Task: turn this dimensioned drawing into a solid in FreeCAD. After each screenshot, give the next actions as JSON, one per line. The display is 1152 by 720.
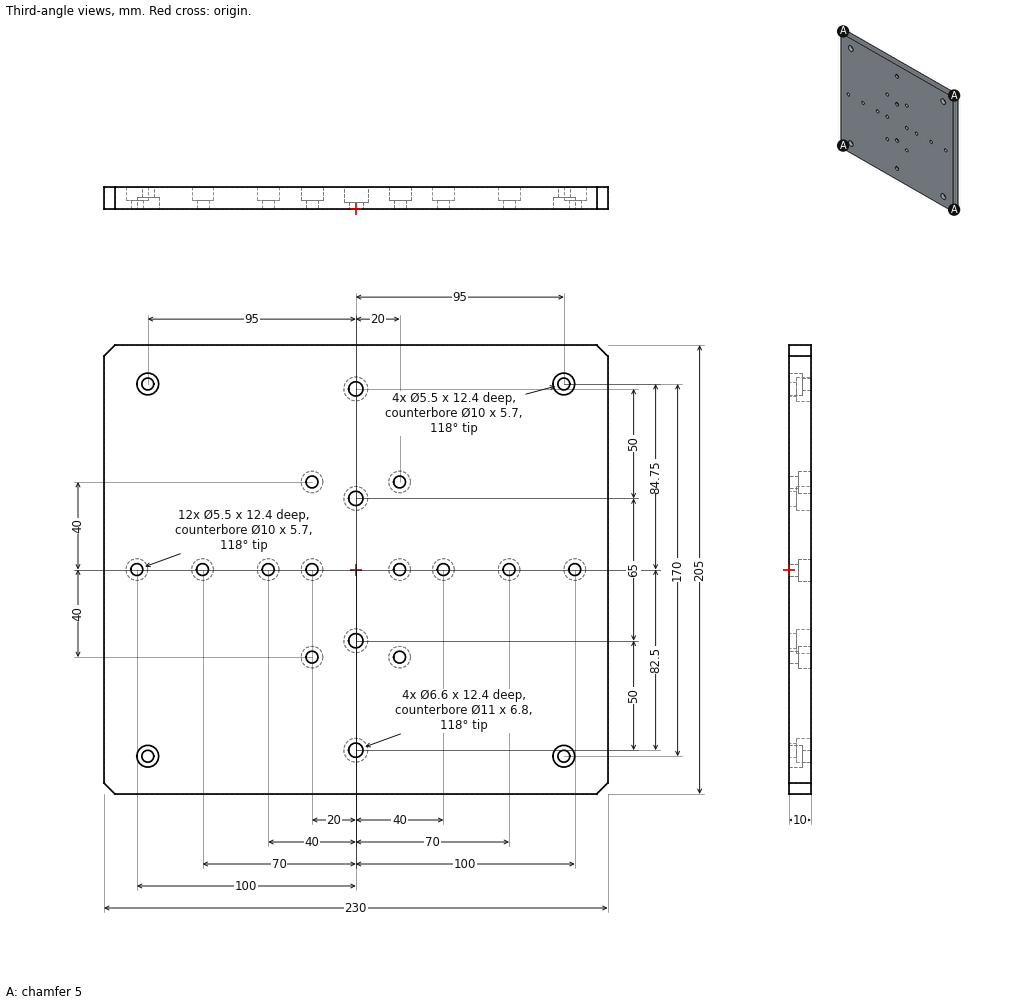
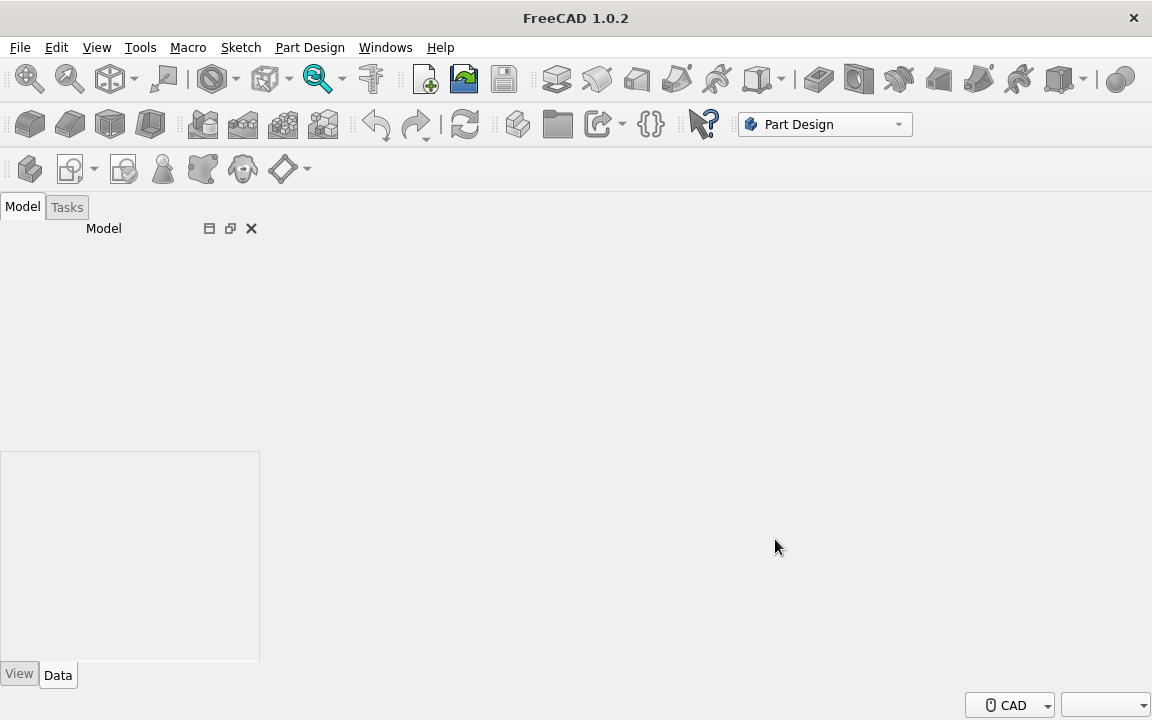
{"action": "left_click", "coordinate": [424, 80]}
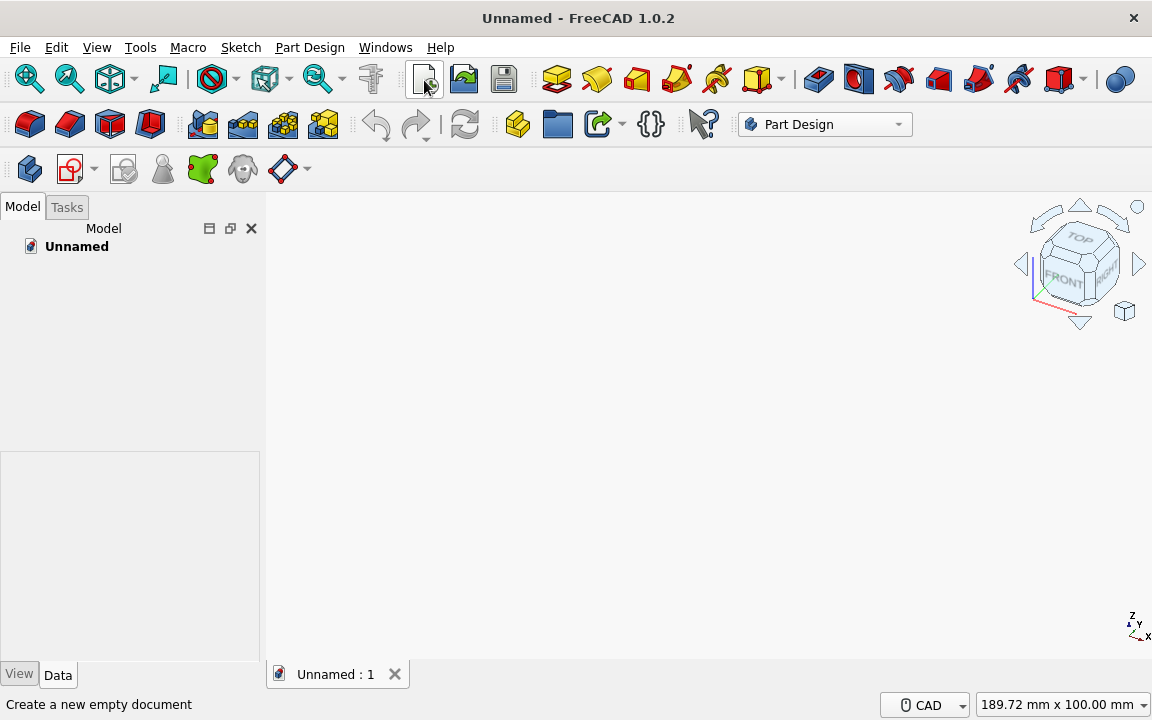
{"action": "left_click", "coordinate": [70, 170]}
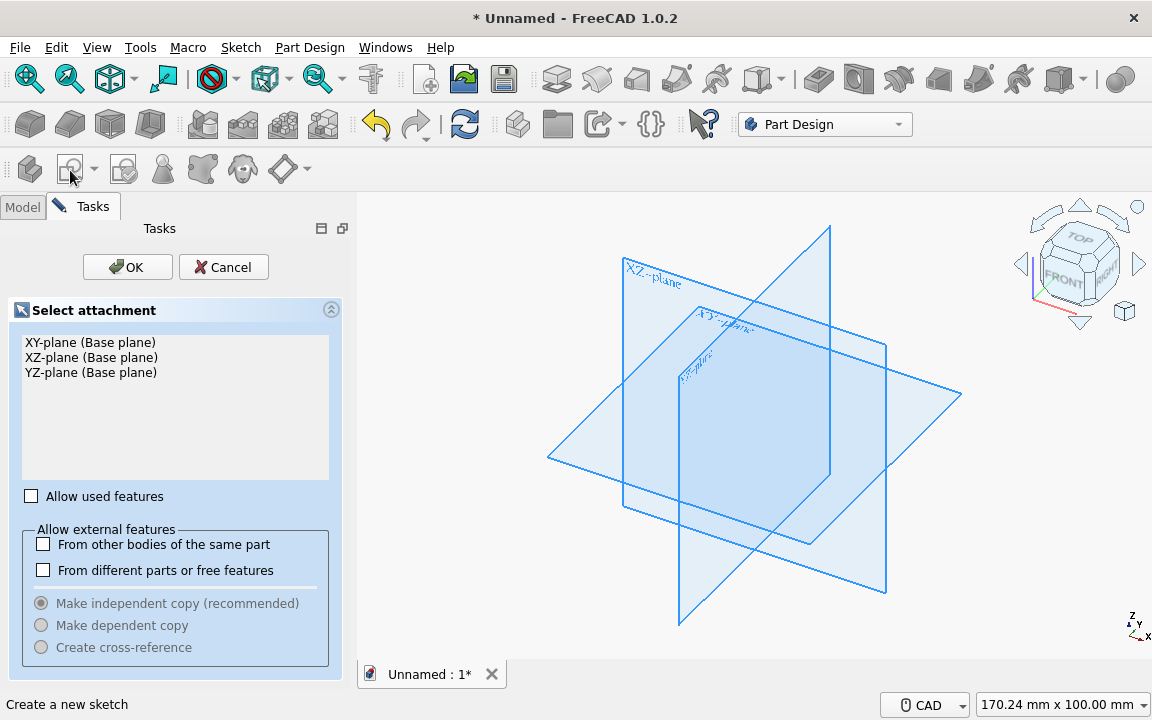
{"action": "left_click", "coordinate": [82, 358]}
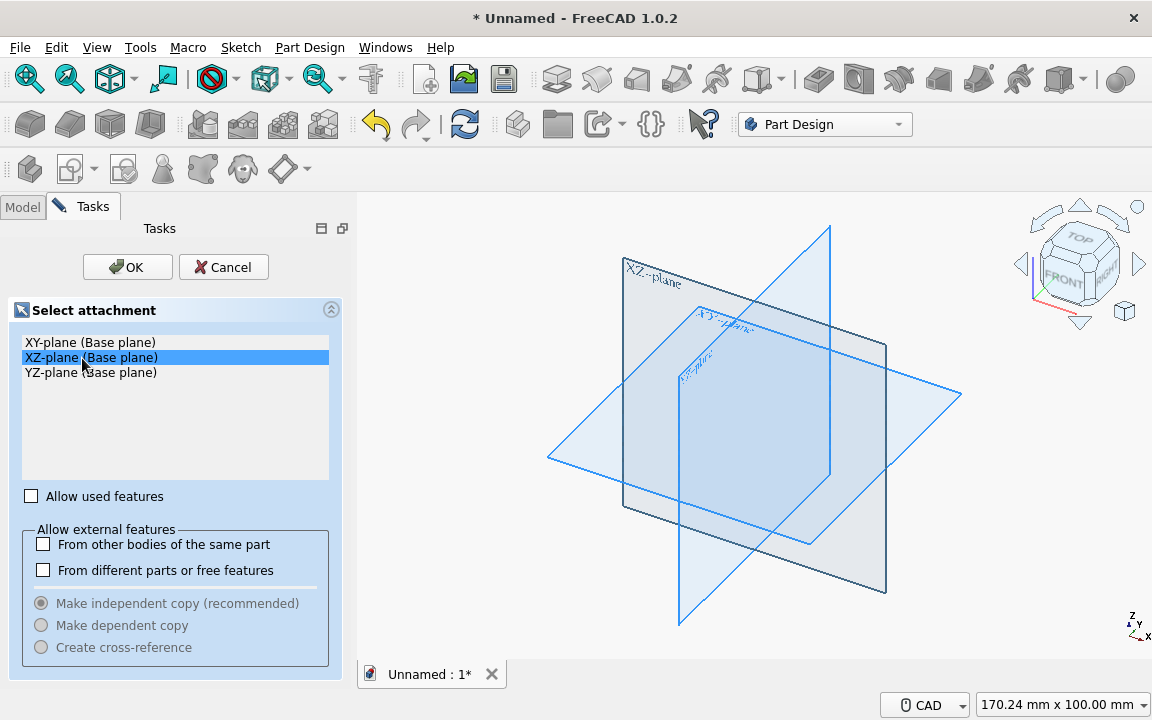
{"action": "left_click", "coordinate": [128, 267]}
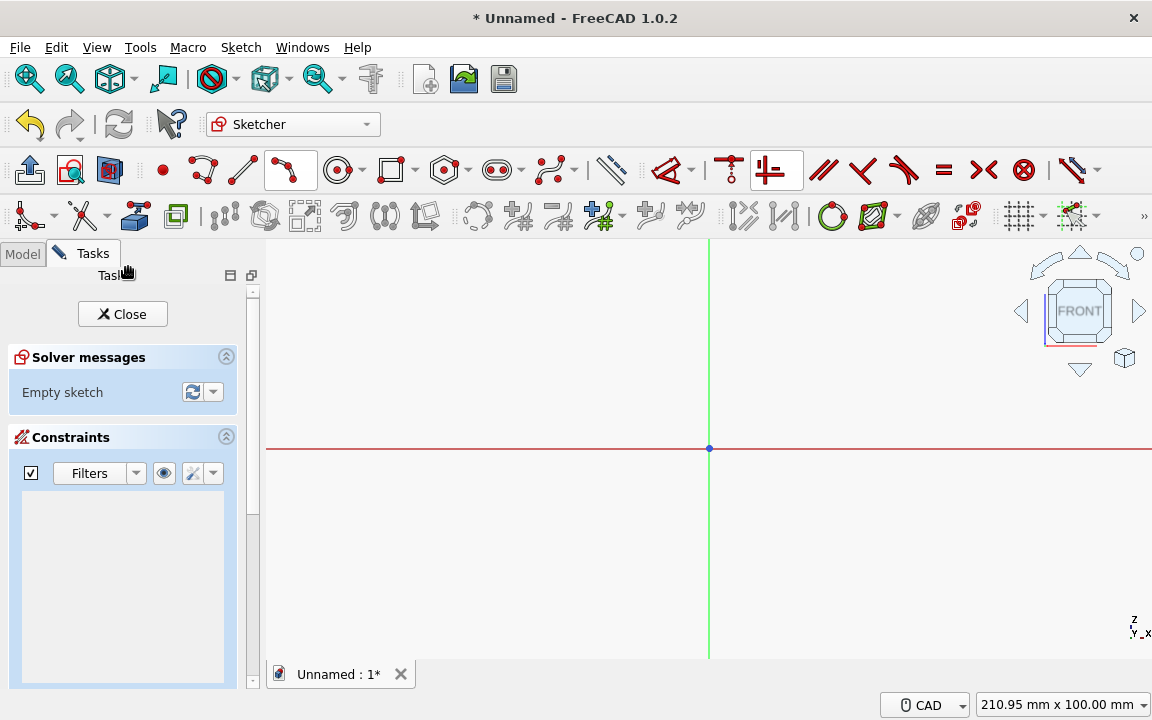
{"action": "scroll", "coordinate": [611, 449], "scroll_direction": "down", "scroll_amount": 6}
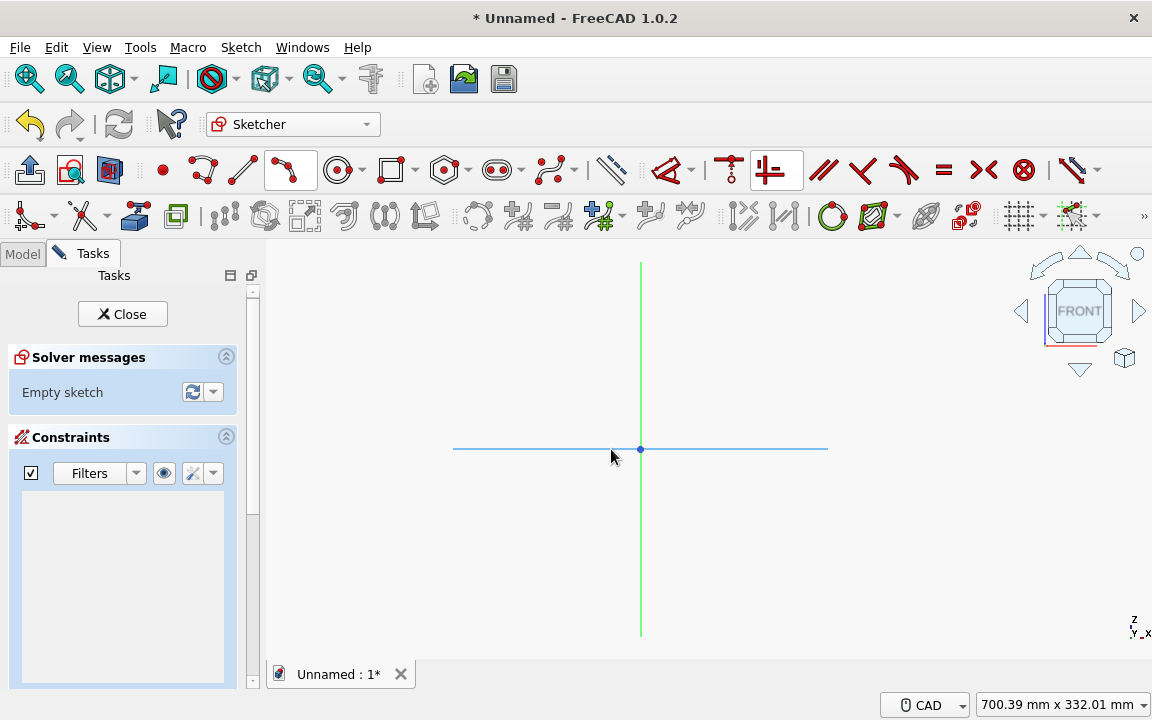
{"action": "key", "text": "g v"}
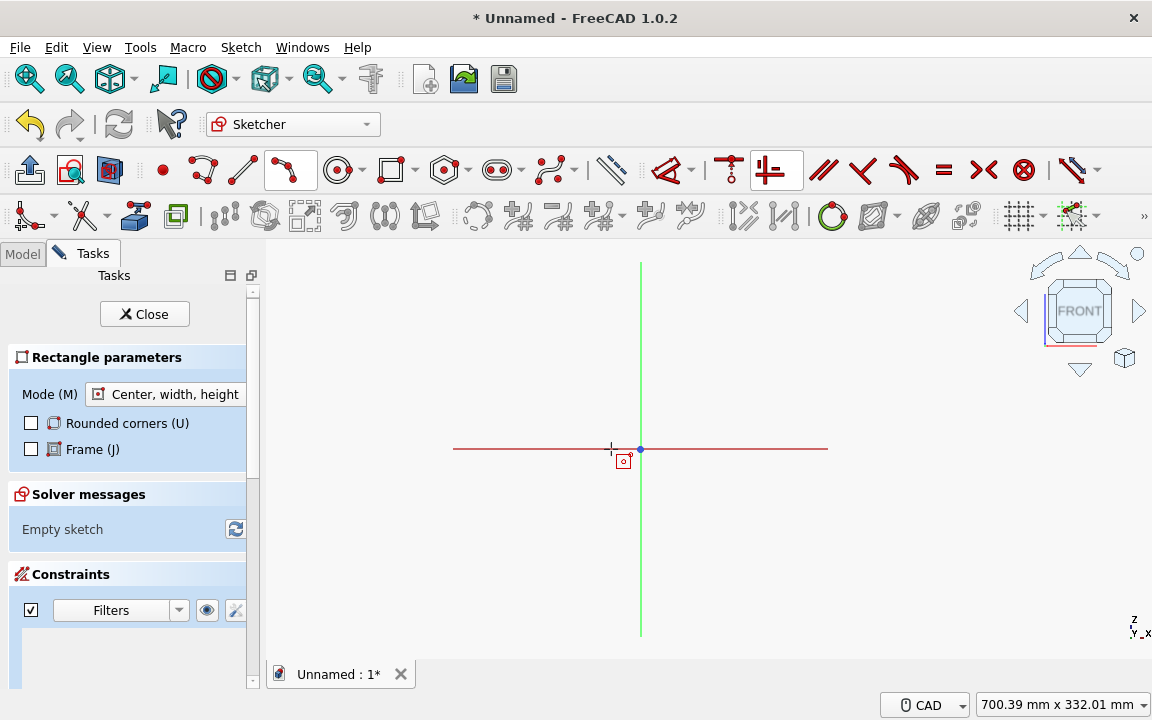
{"action": "left_click", "coordinate": [641, 449]}
{"action": "left_click", "coordinate": [786, 320]}
{"action": "key", "text": "Escape"}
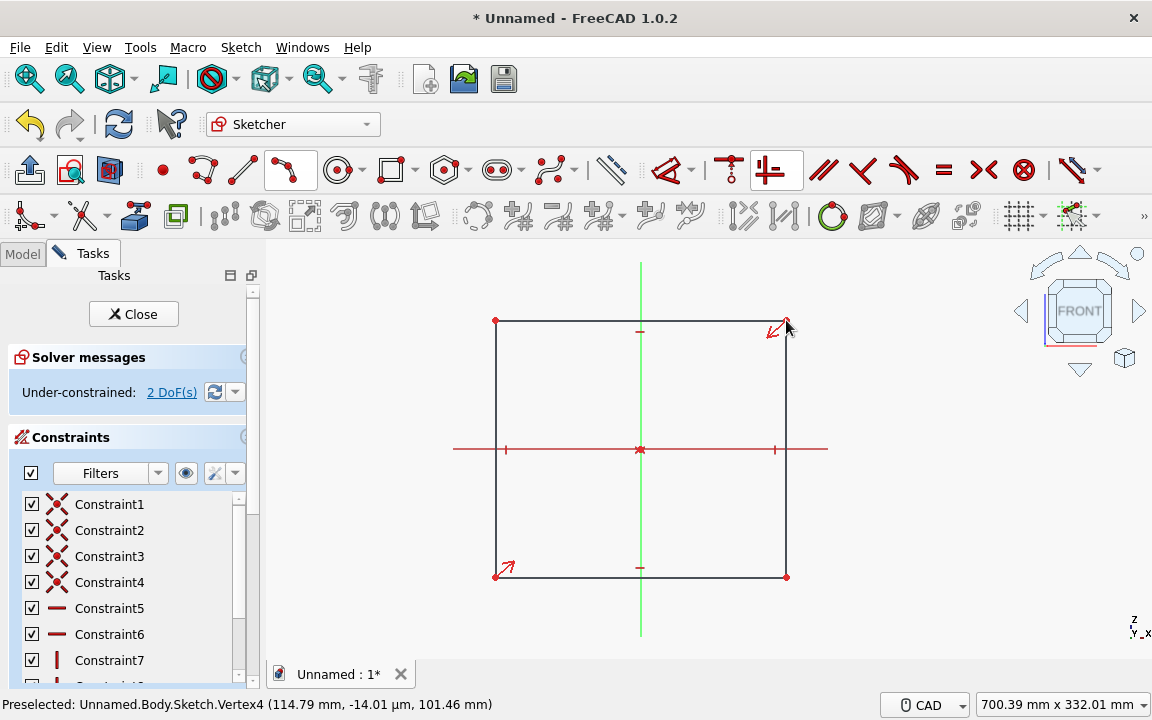
{"action": "left_click", "coordinate": [666, 170]}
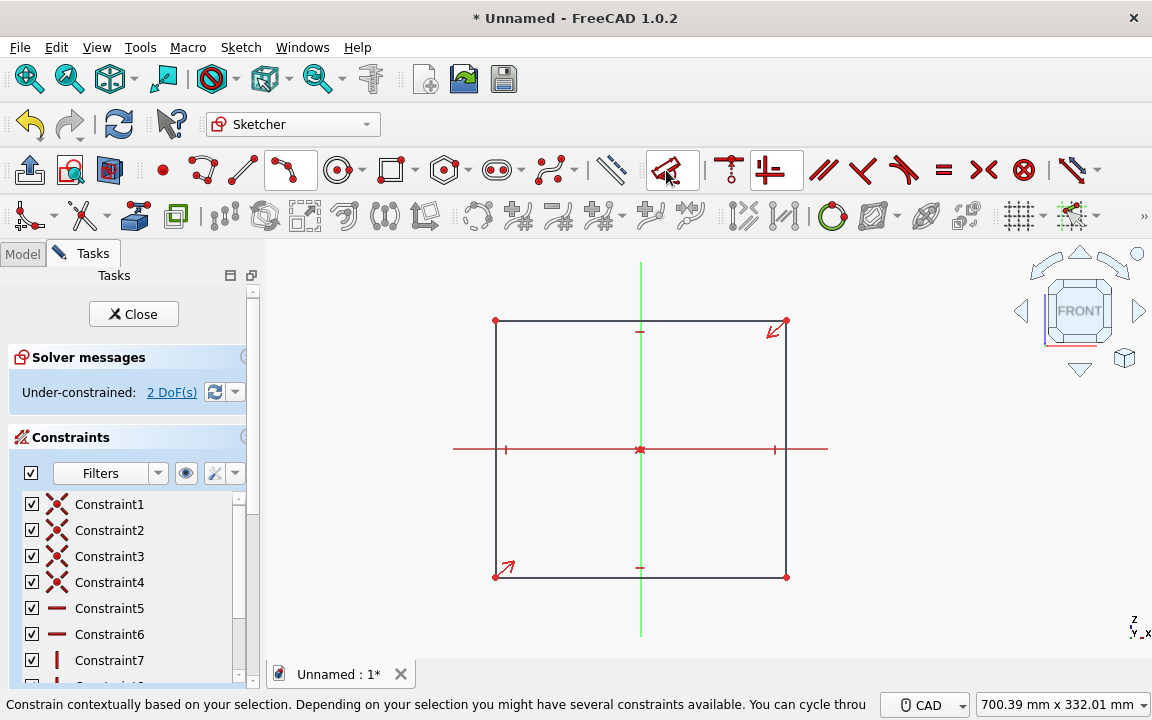
{"action": "left_click", "coordinate": [583, 578]}
{"action": "left_click", "coordinate": [574, 612]}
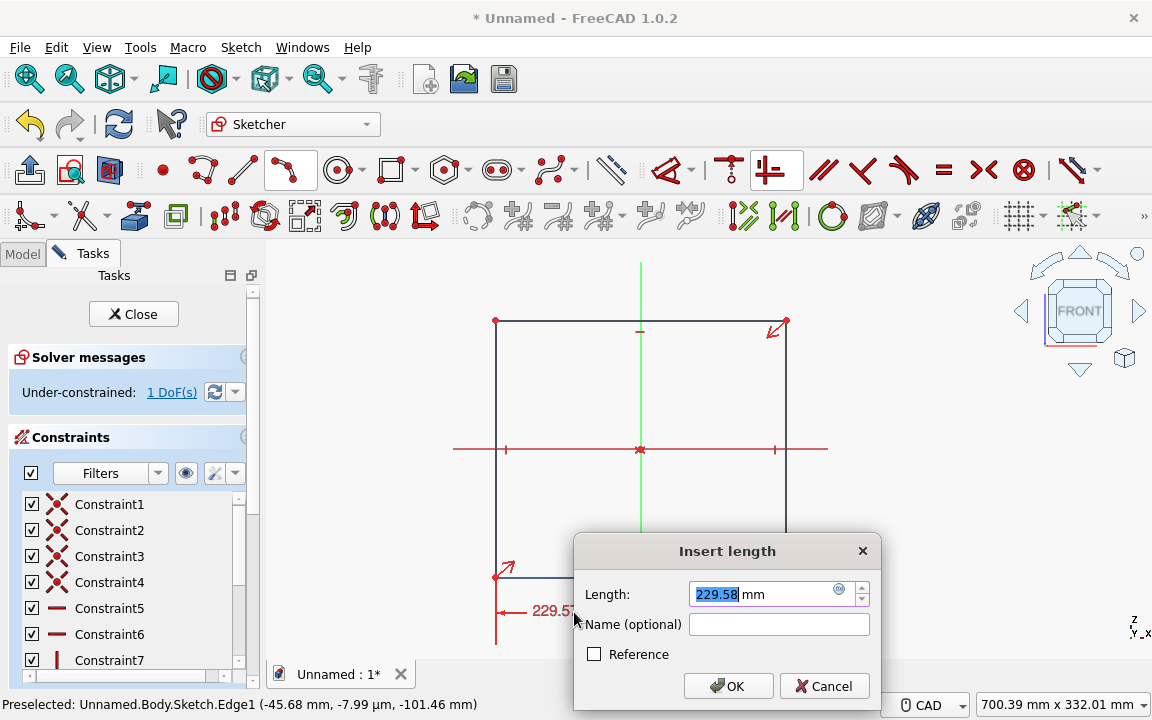
{"action": "type", "text": "230"}
{"action": "key", "text": "Return"}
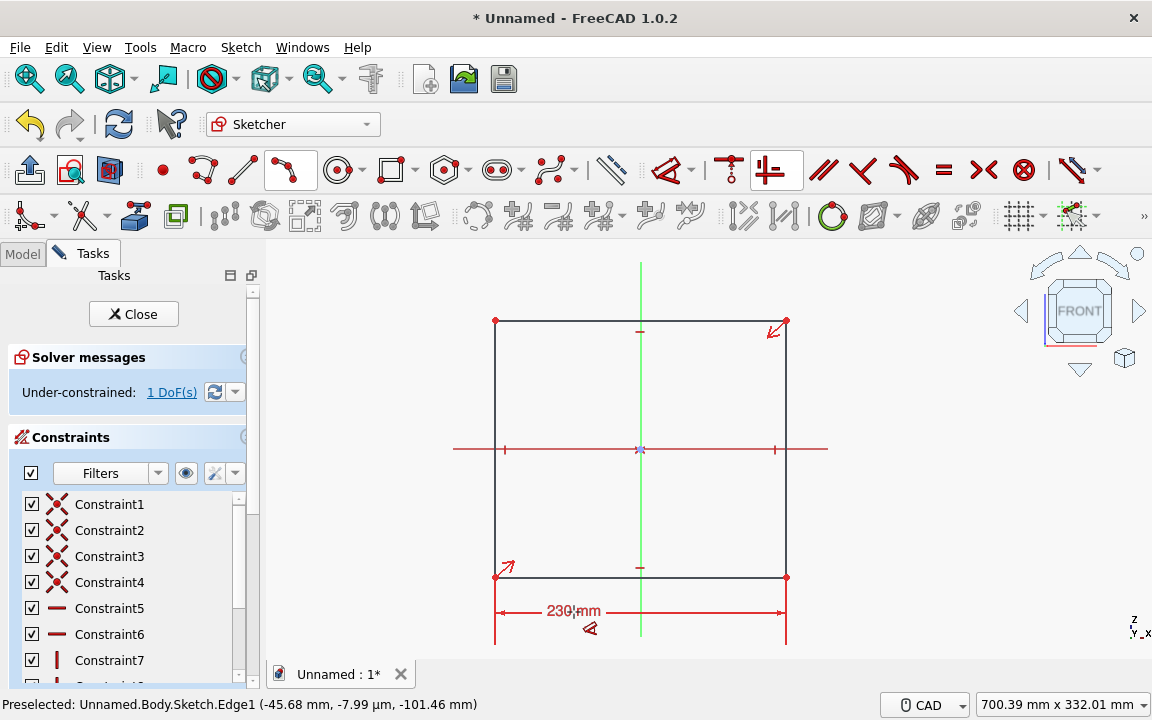
{"action": "left_click", "coordinate": [786, 501]}
{"action": "left_click", "coordinate": [820, 390]}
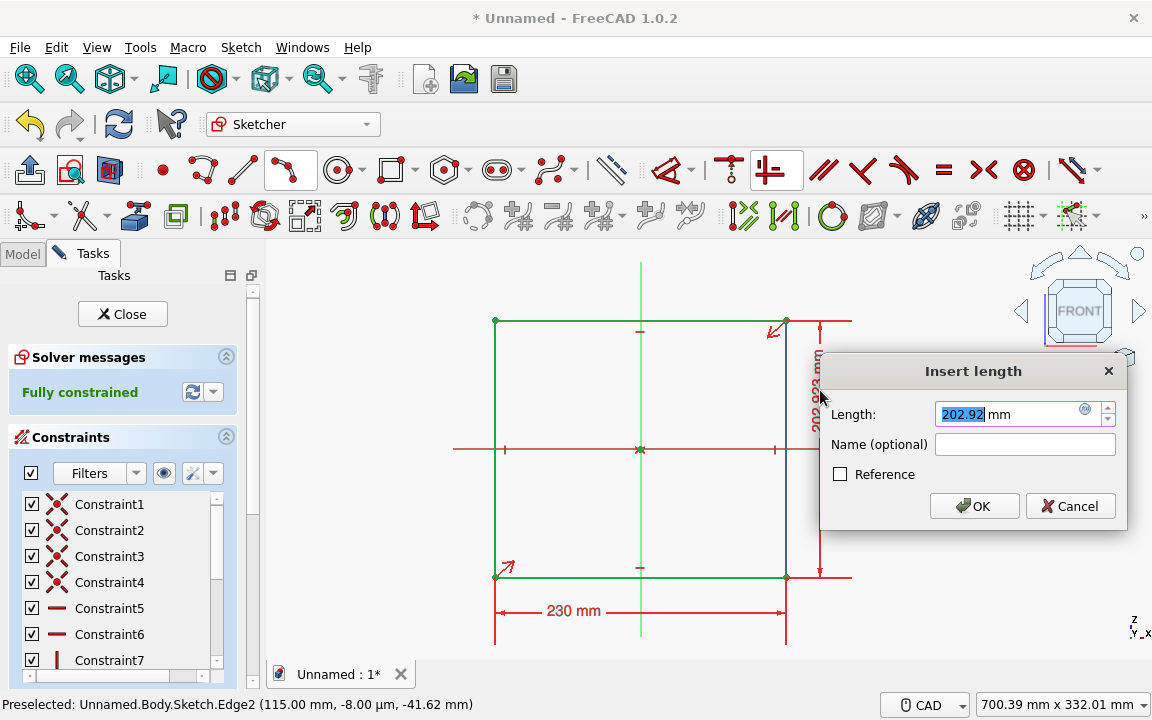
{"action": "type", "text": "205"}
{"action": "key", "text": "Return"}
{"action": "key", "text": "Escape"}